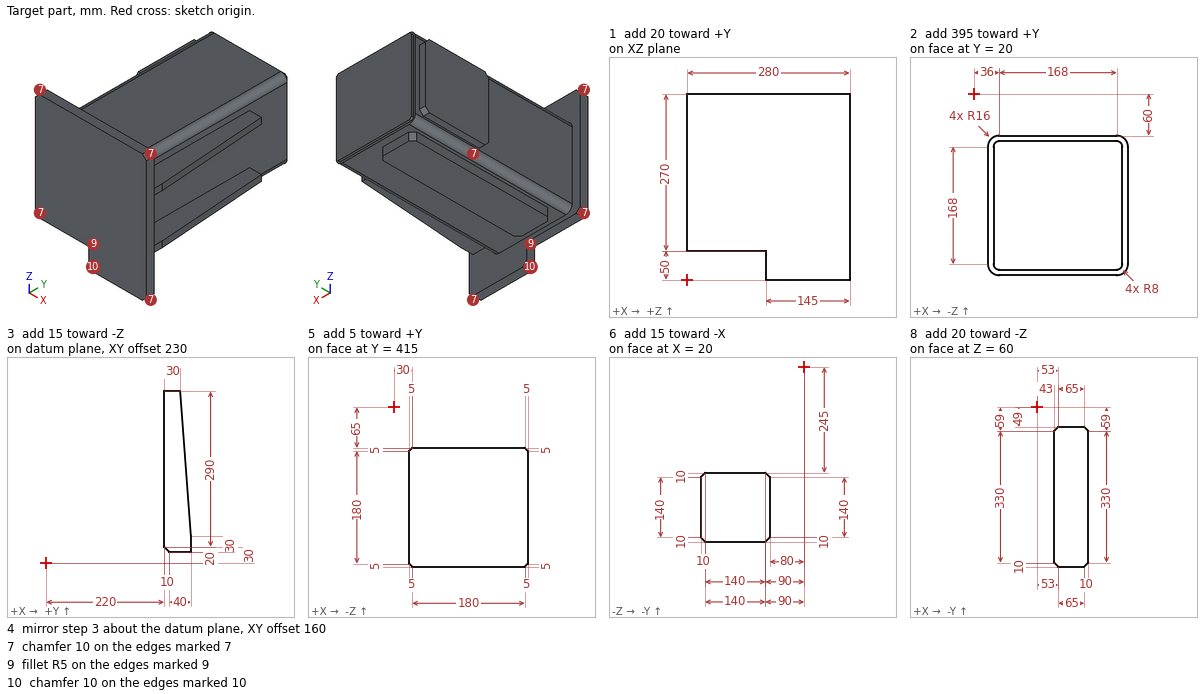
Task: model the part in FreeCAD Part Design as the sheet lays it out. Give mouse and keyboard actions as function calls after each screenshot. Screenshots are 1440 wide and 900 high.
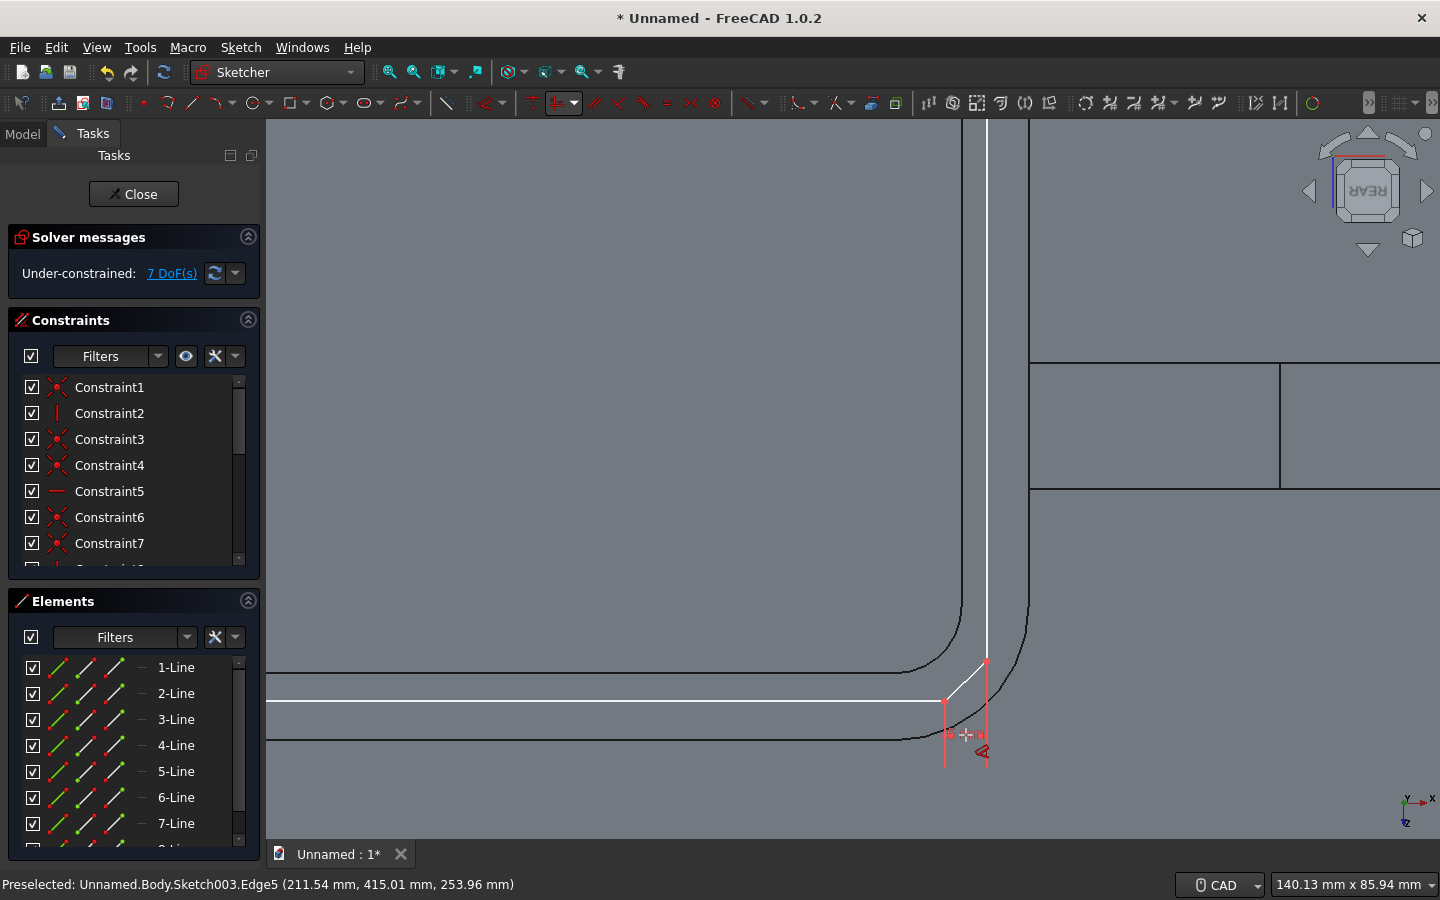
click(957, 689)
click(1021, 681)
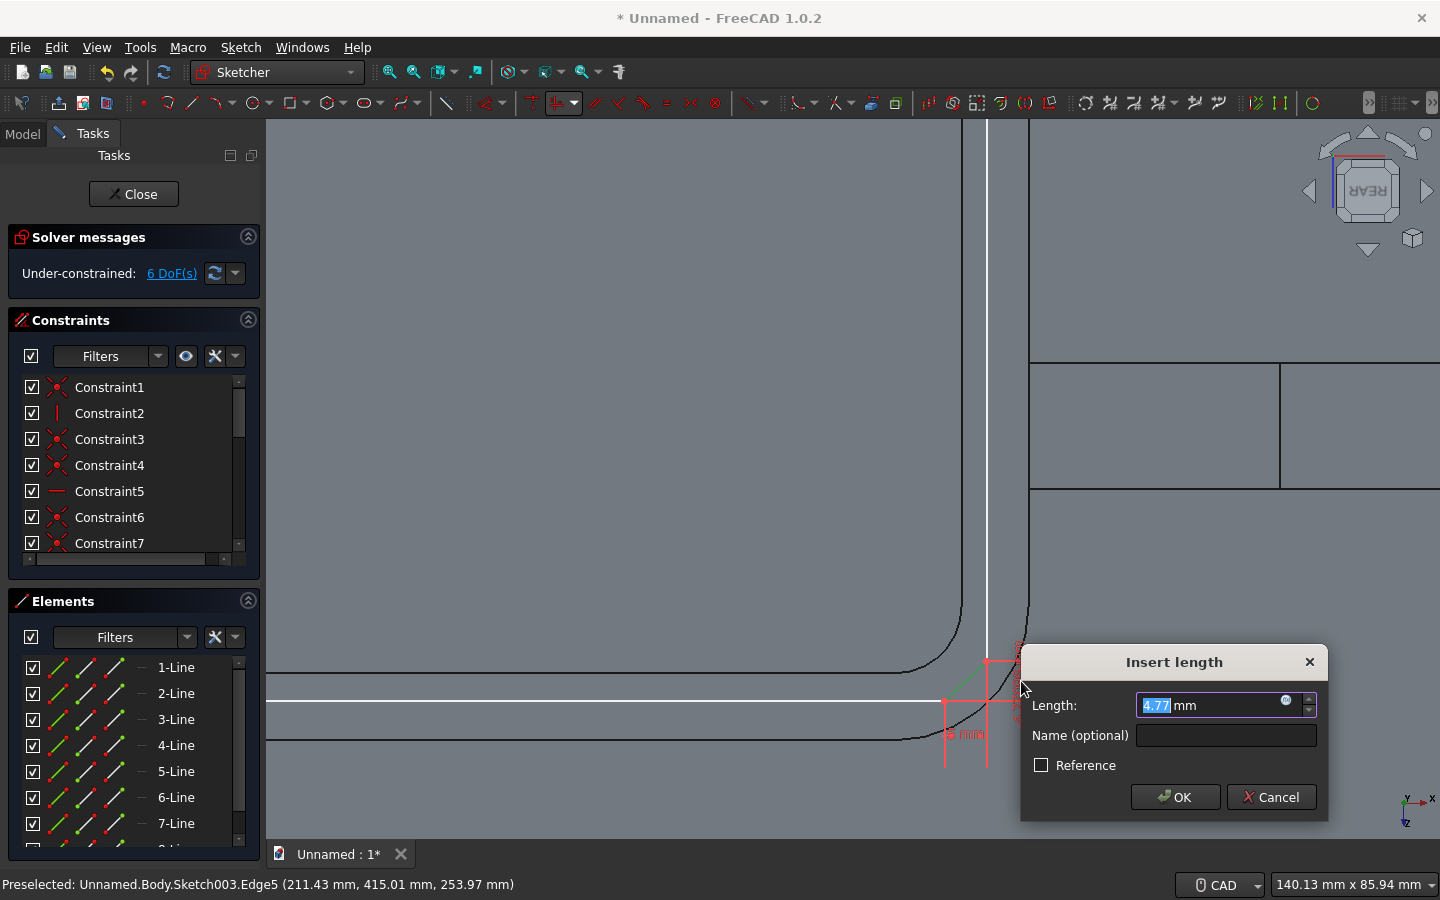
text(5)
key(Return)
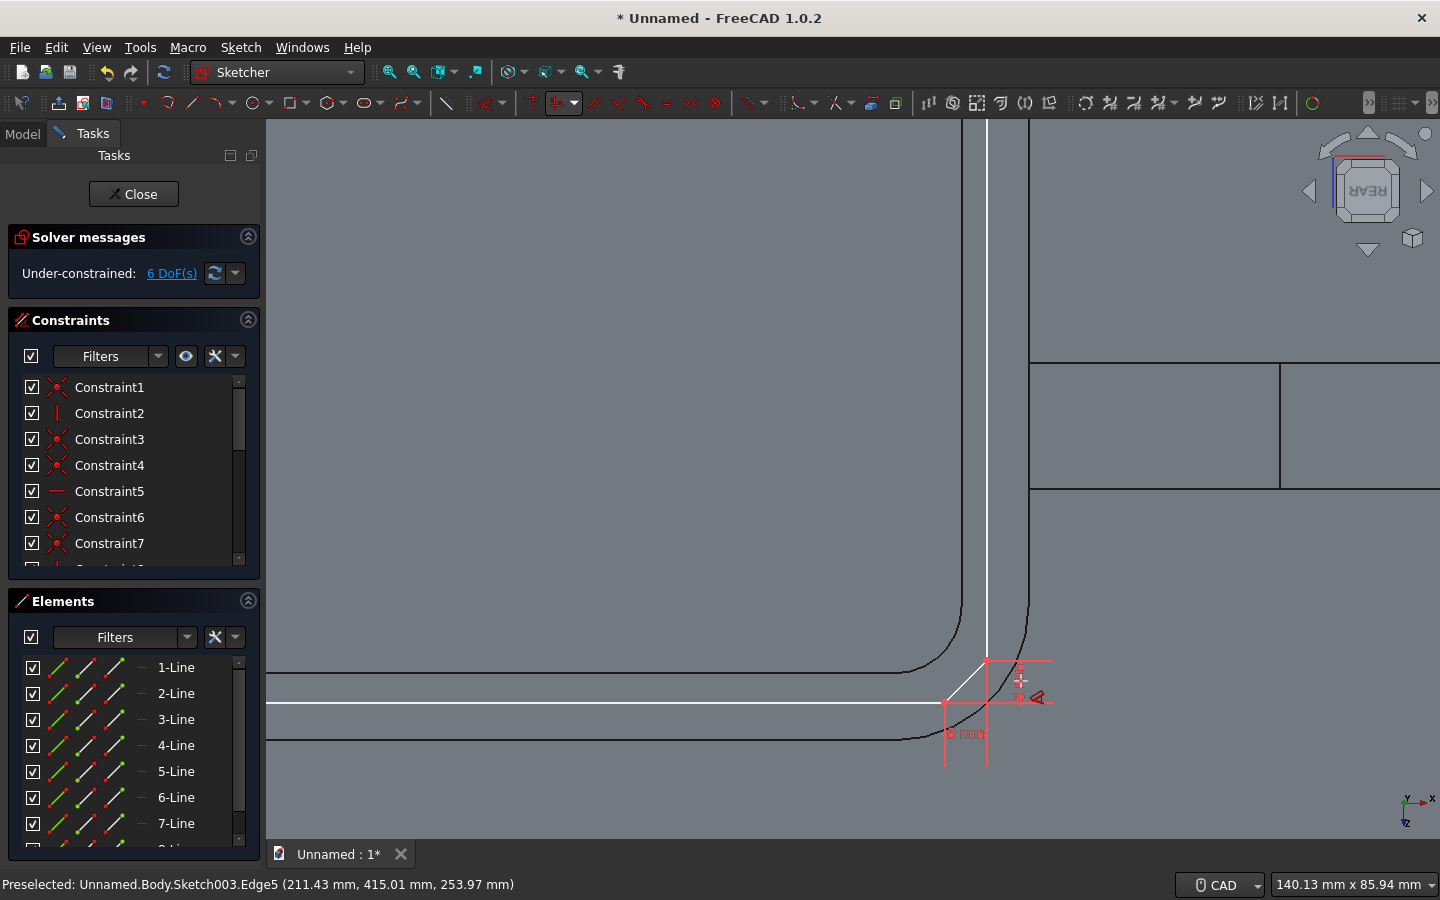
scroll(961, 694, down, 8)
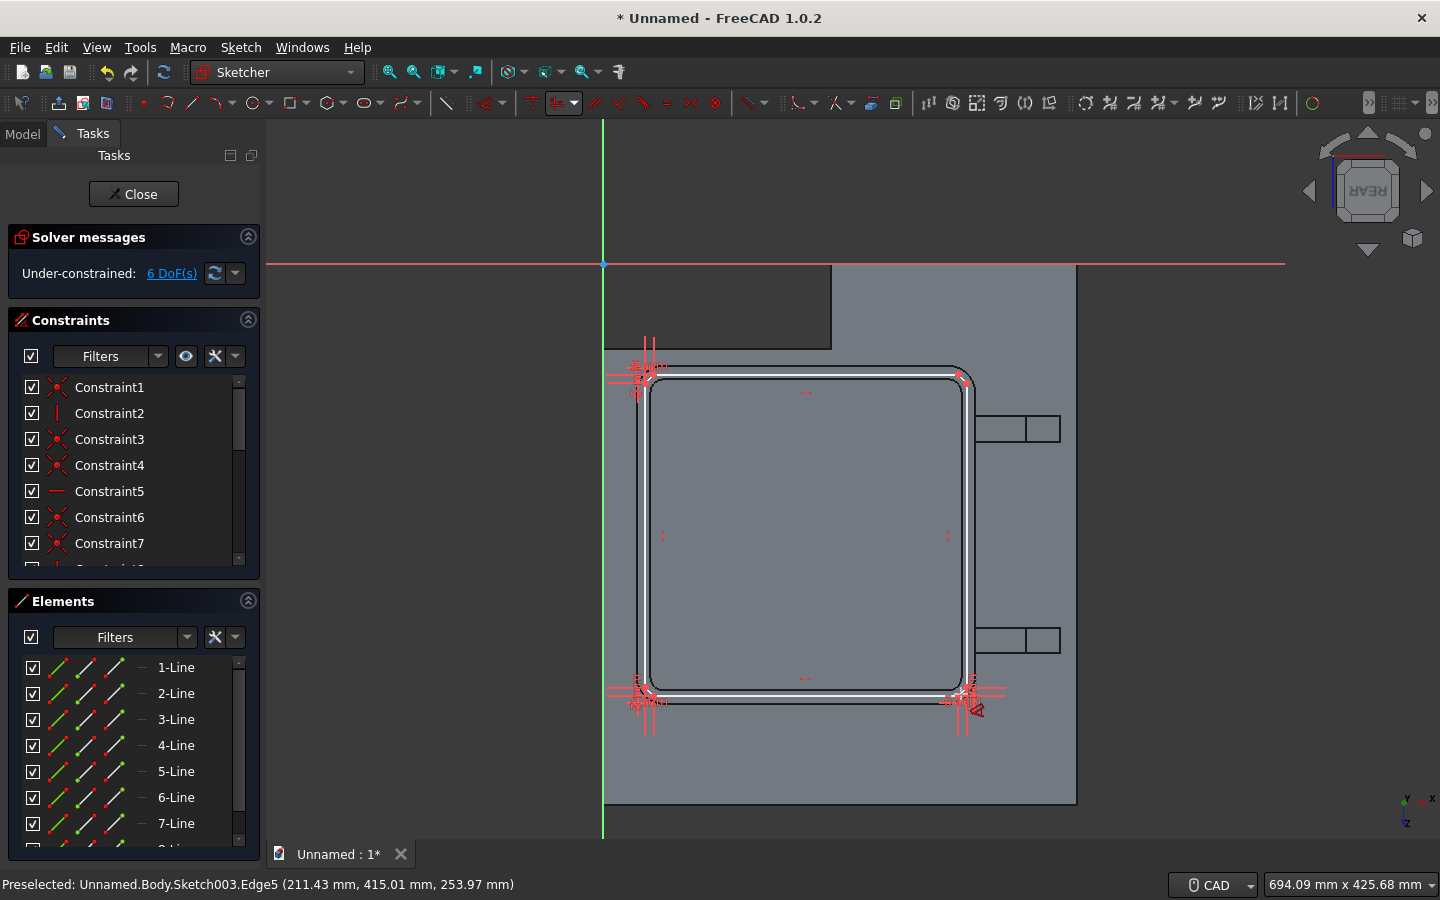
scroll(964, 381, up, 8)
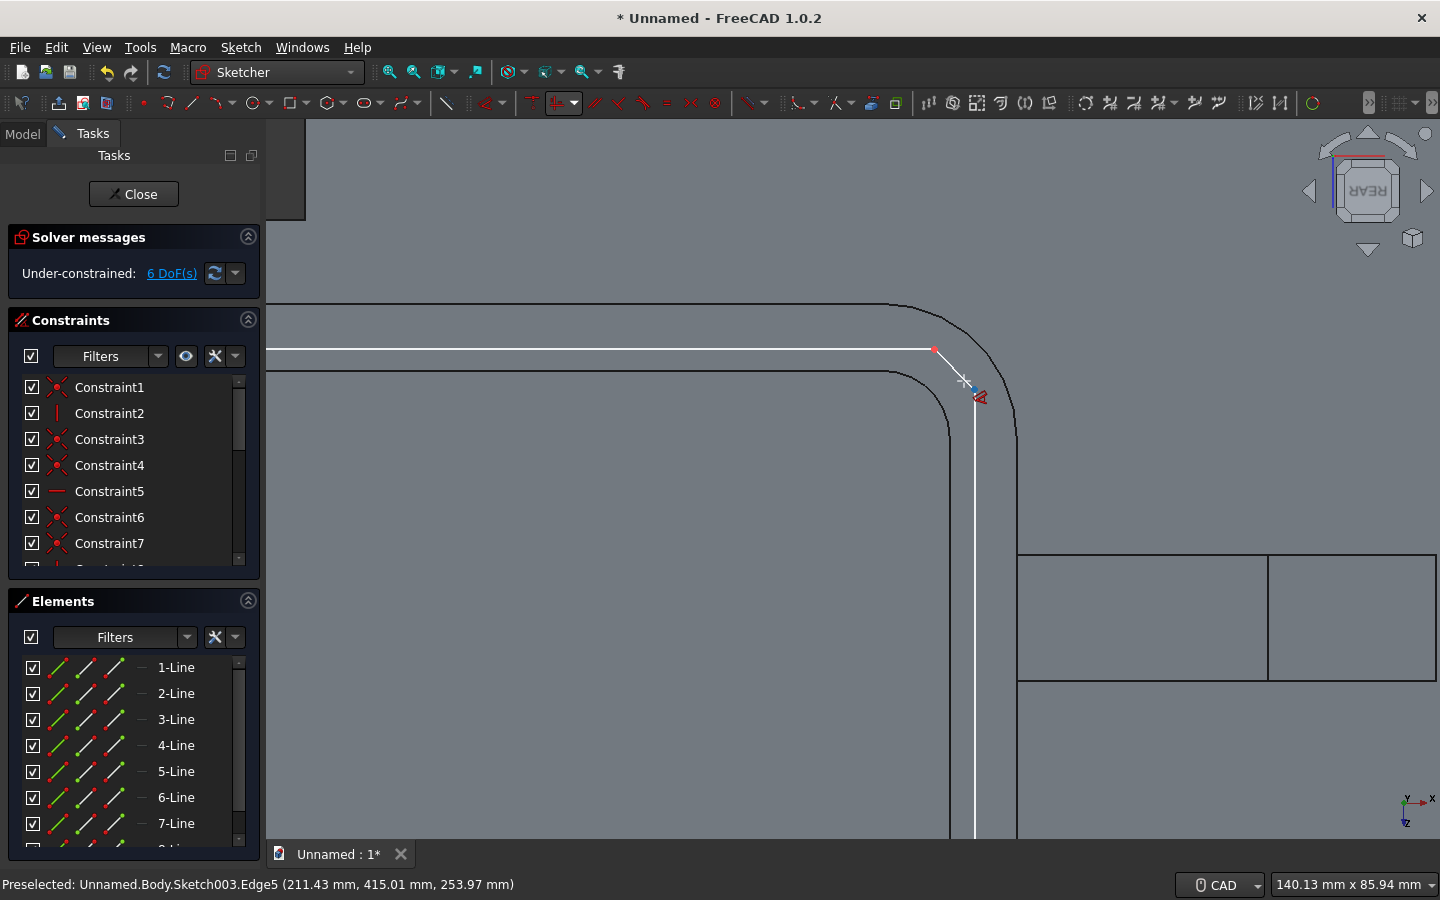
click(963, 378)
click(954, 315)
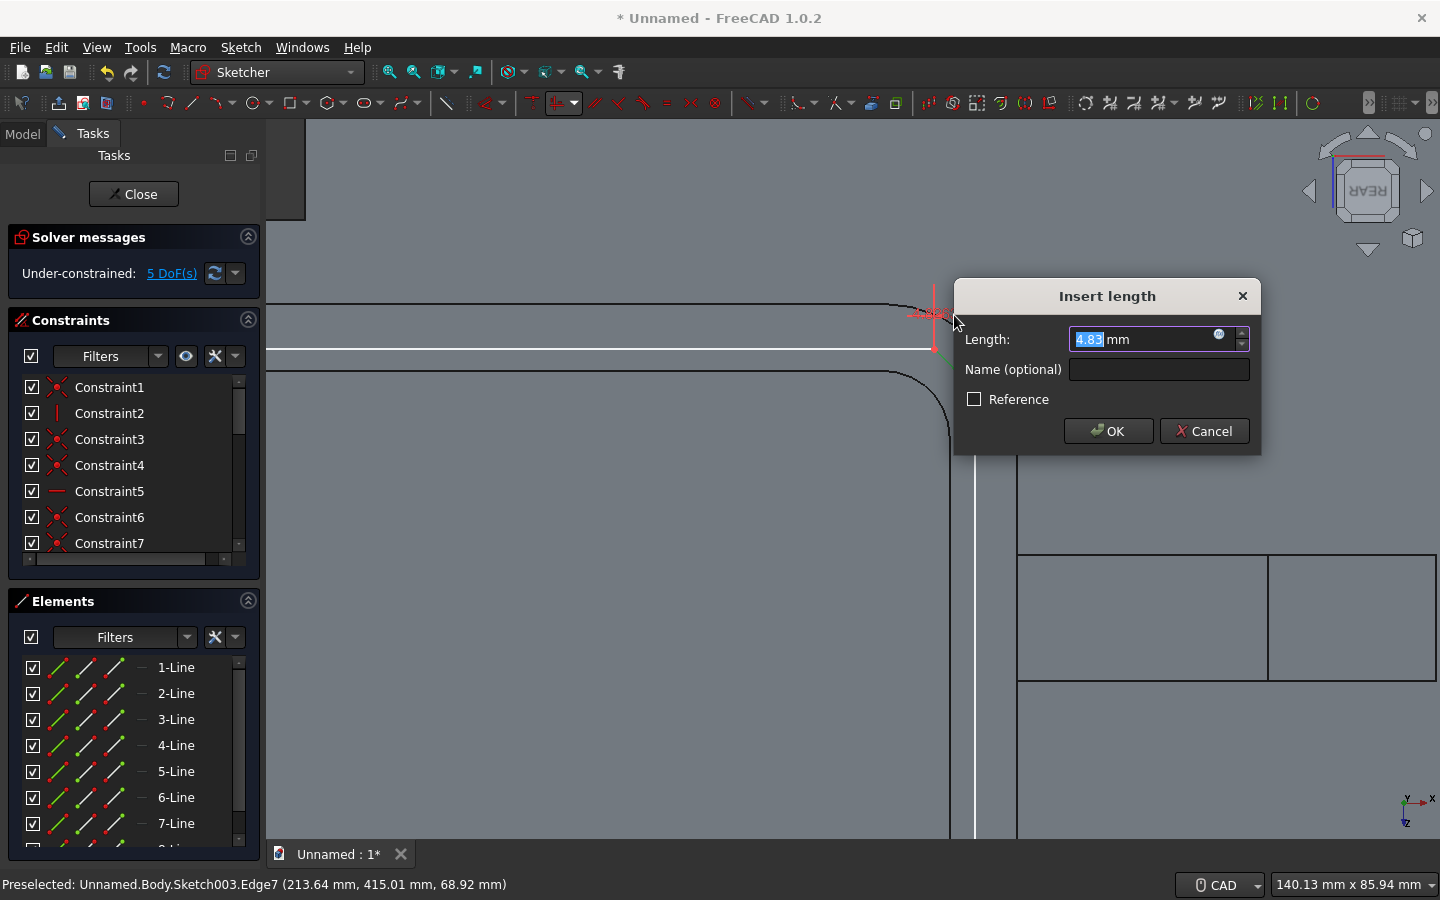
text(5)
key(Return)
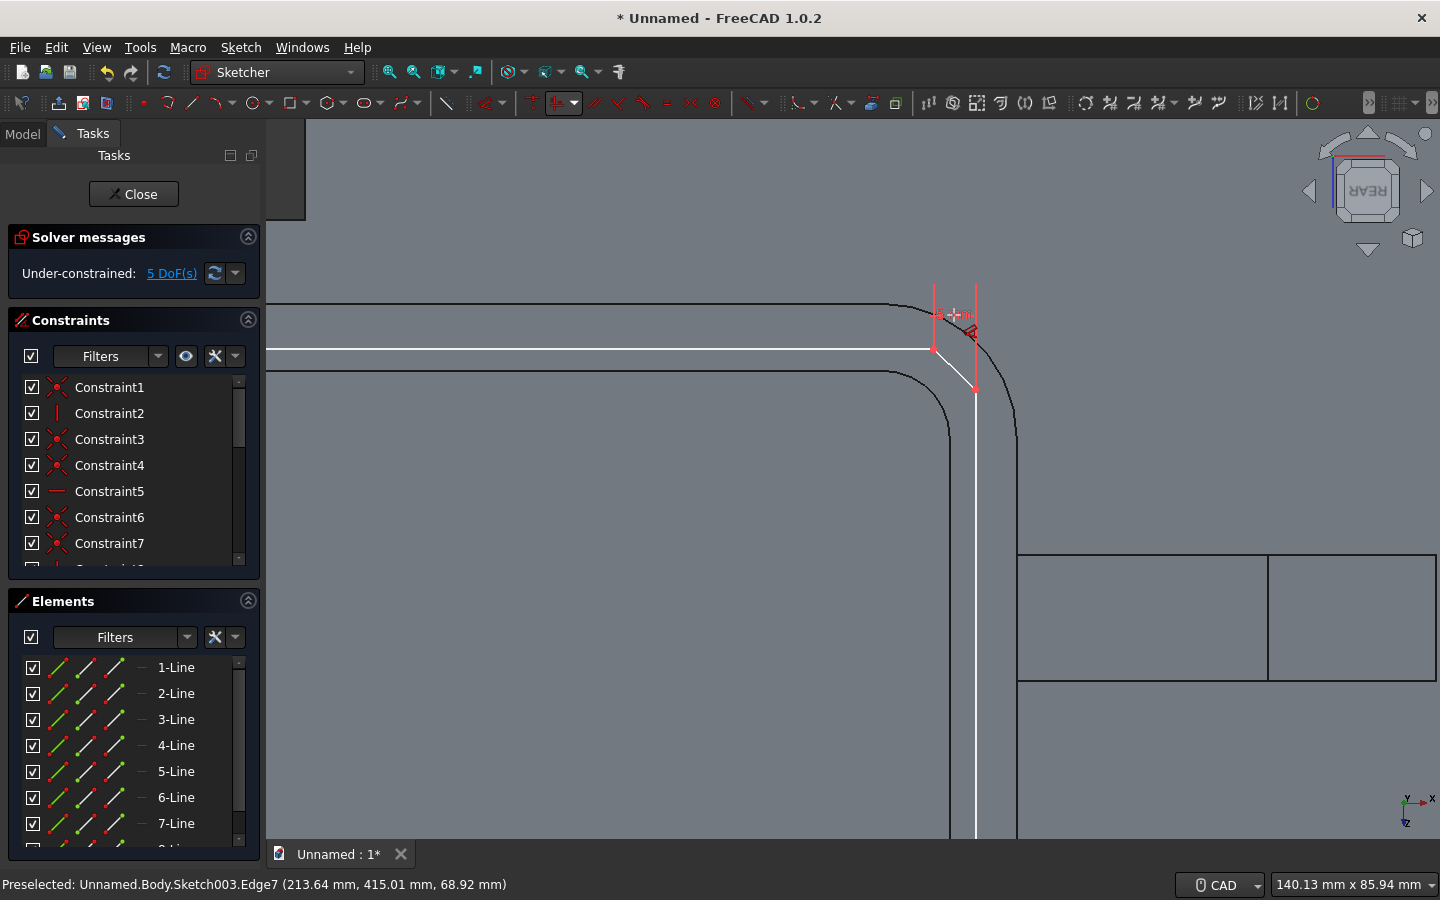
click(963, 378)
click(1010, 369)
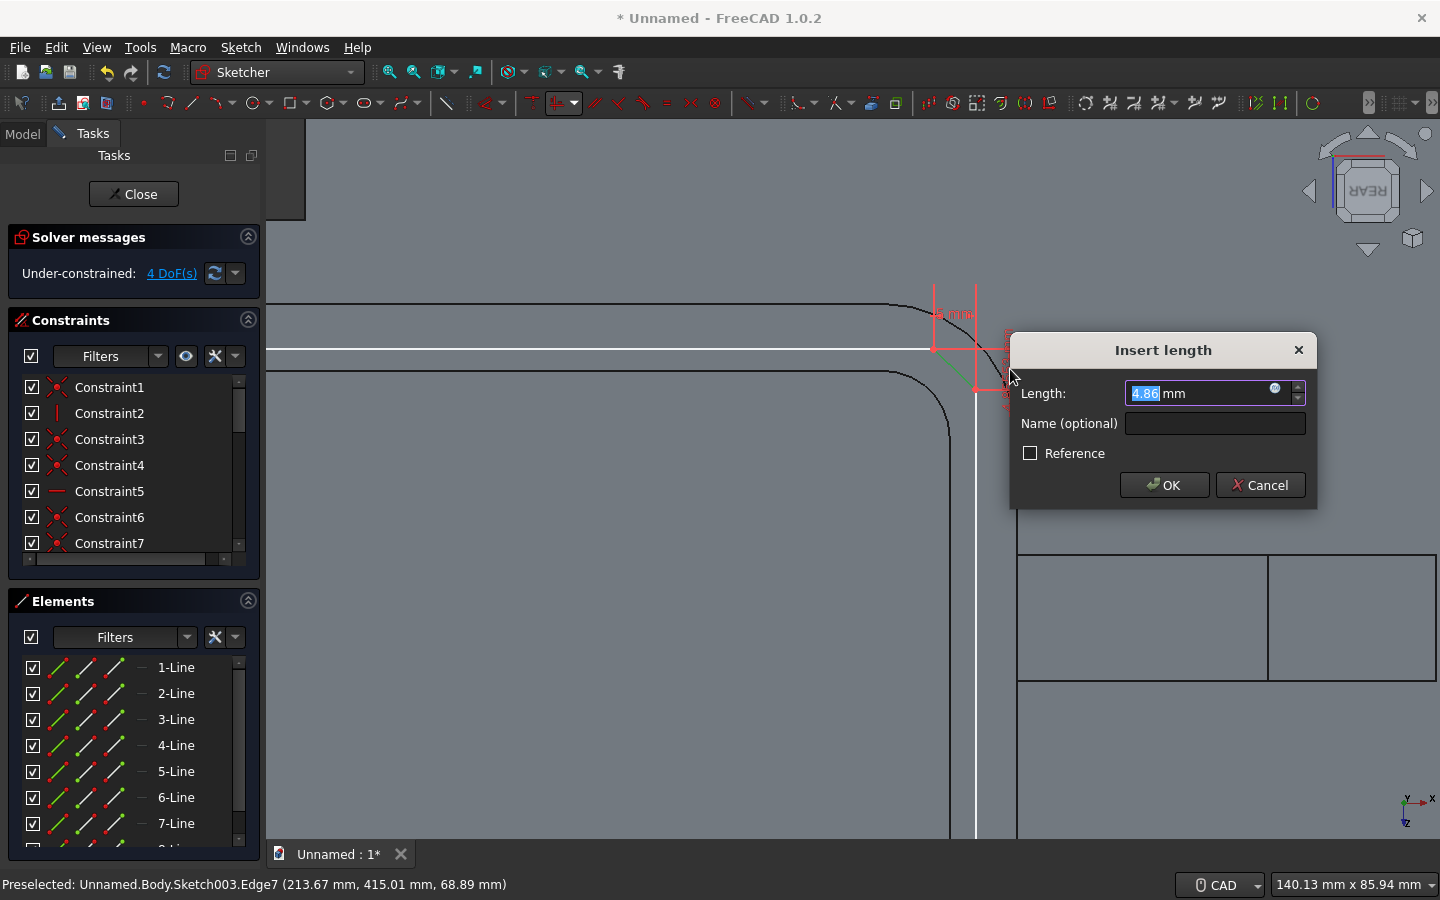
text(5)
key(Return)